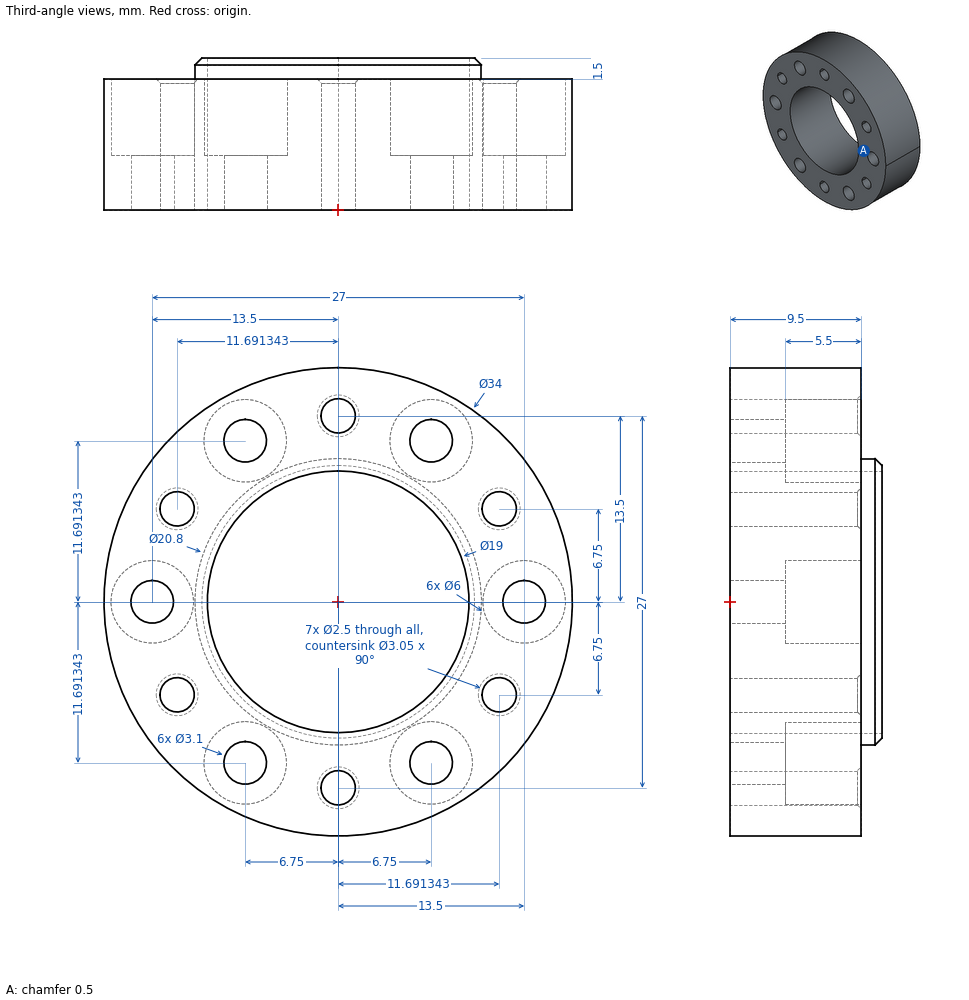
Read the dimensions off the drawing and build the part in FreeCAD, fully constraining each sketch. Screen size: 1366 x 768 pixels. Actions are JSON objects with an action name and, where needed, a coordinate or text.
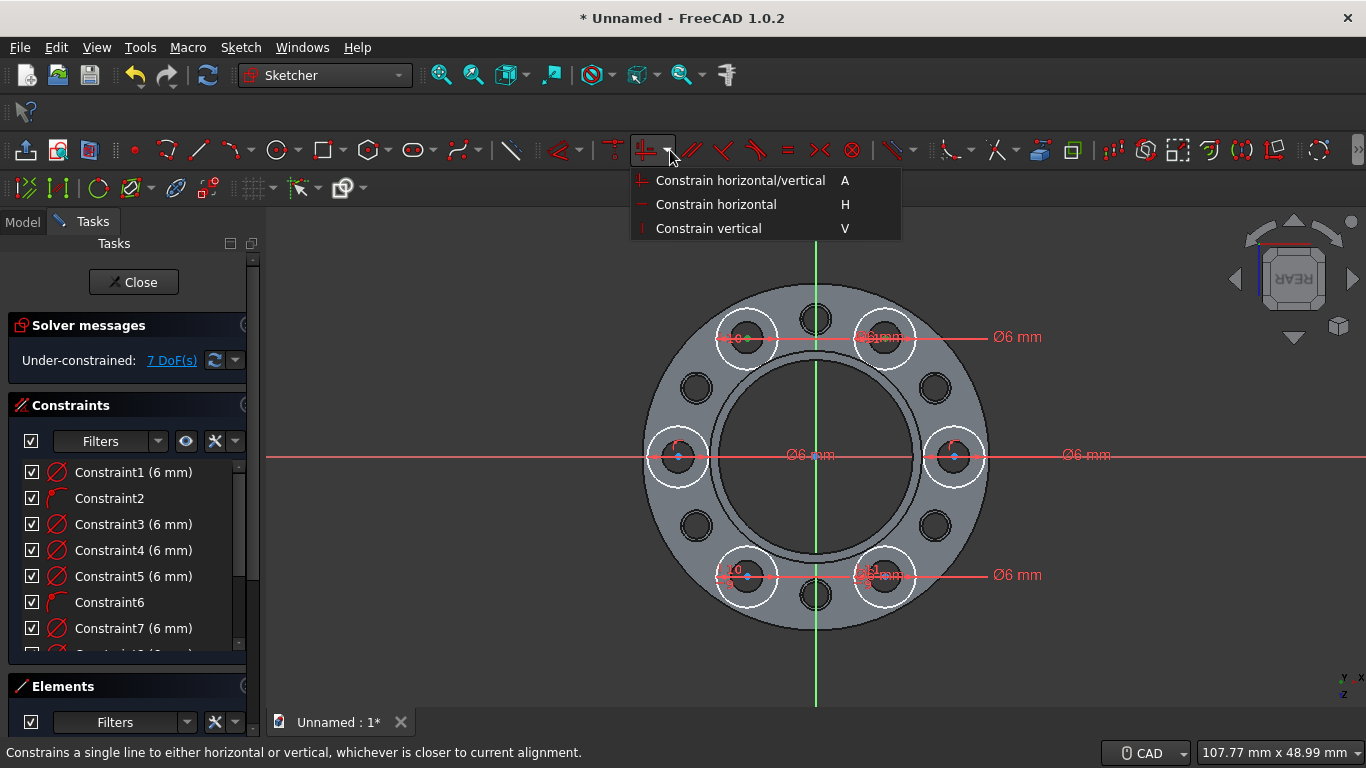
{"action": "left_click", "coordinate": [766, 204]}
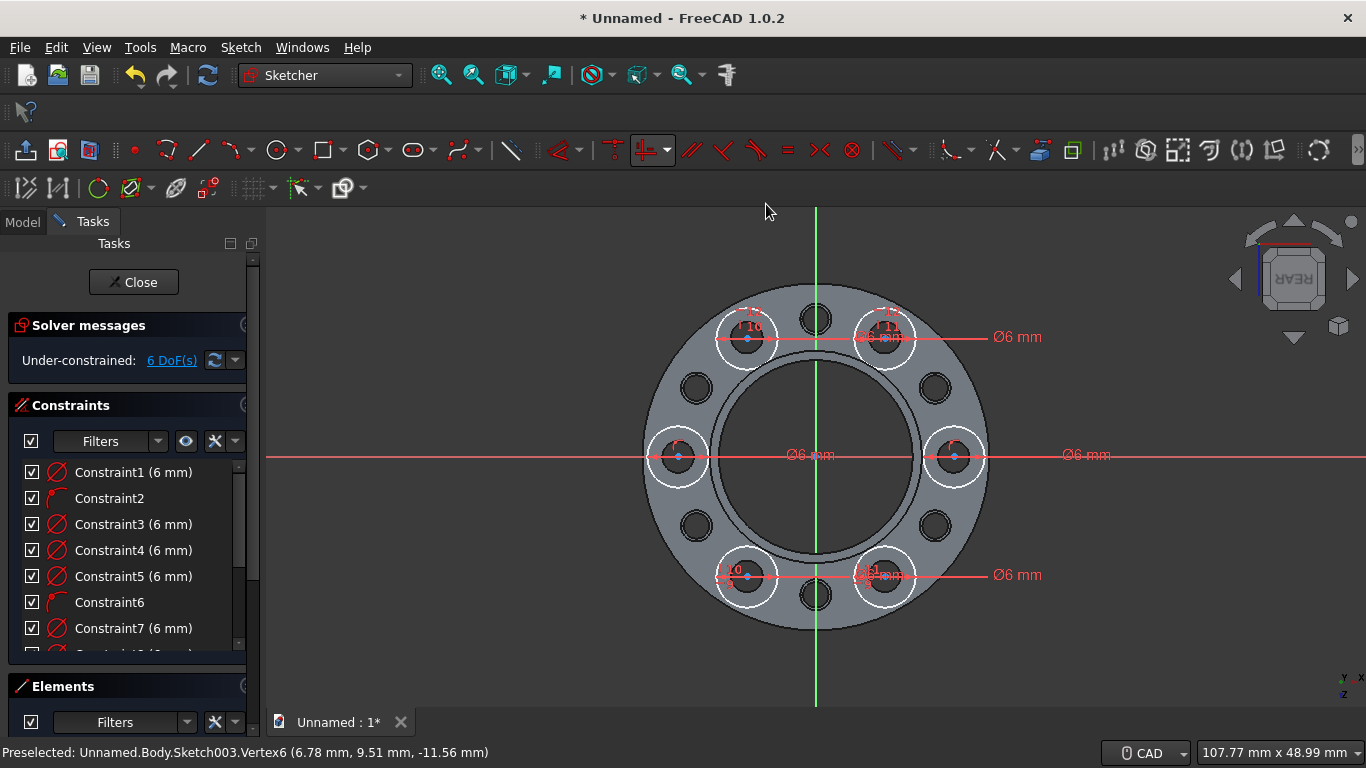
{"action": "left_click", "coordinate": [558, 150]}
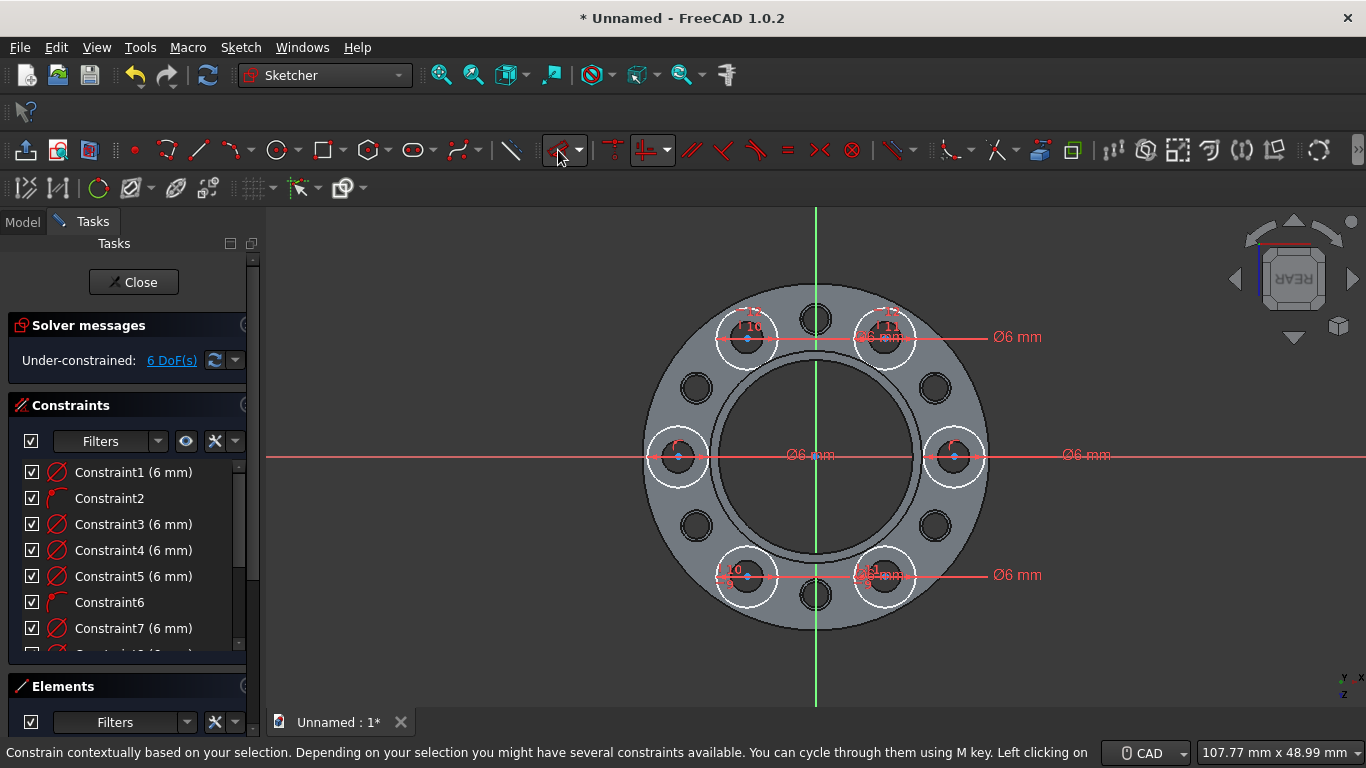
{"action": "left_click", "coordinate": [954, 457]}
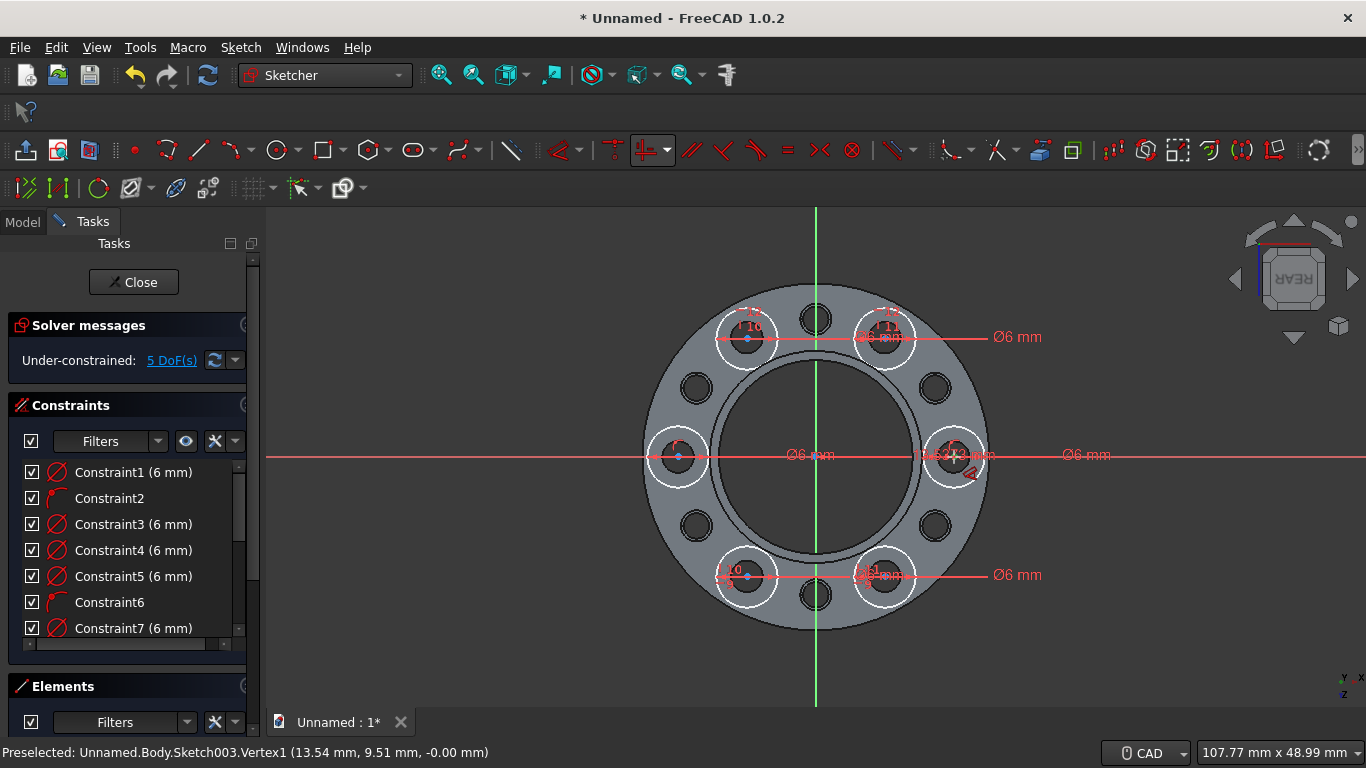
{"action": "left_click", "coordinate": [678, 457]}
{"action": "left_click", "coordinate": [753, 491]}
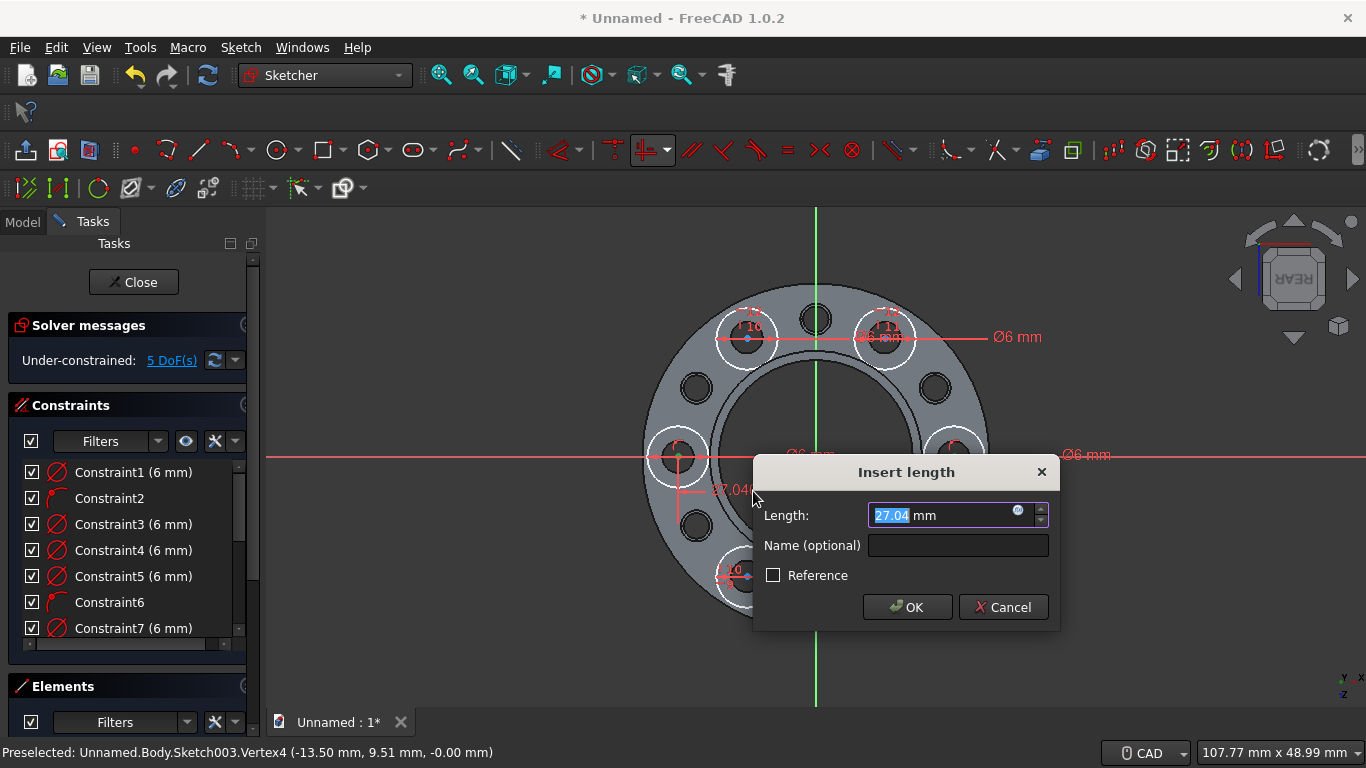
{"action": "type", "text": "27"}
{"action": "key", "text": "Return"}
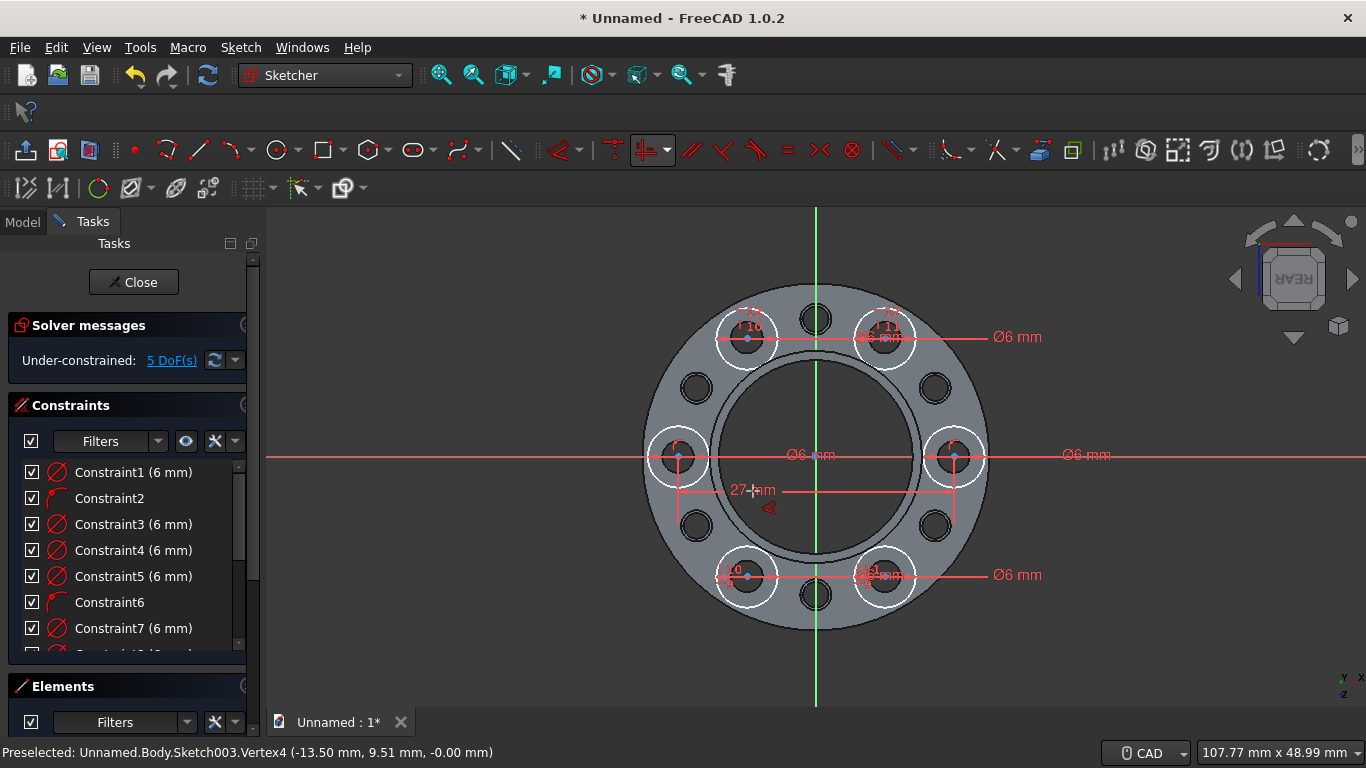
{"action": "left_click", "coordinate": [954, 457]}
{"action": "left_click", "coordinate": [885, 491]}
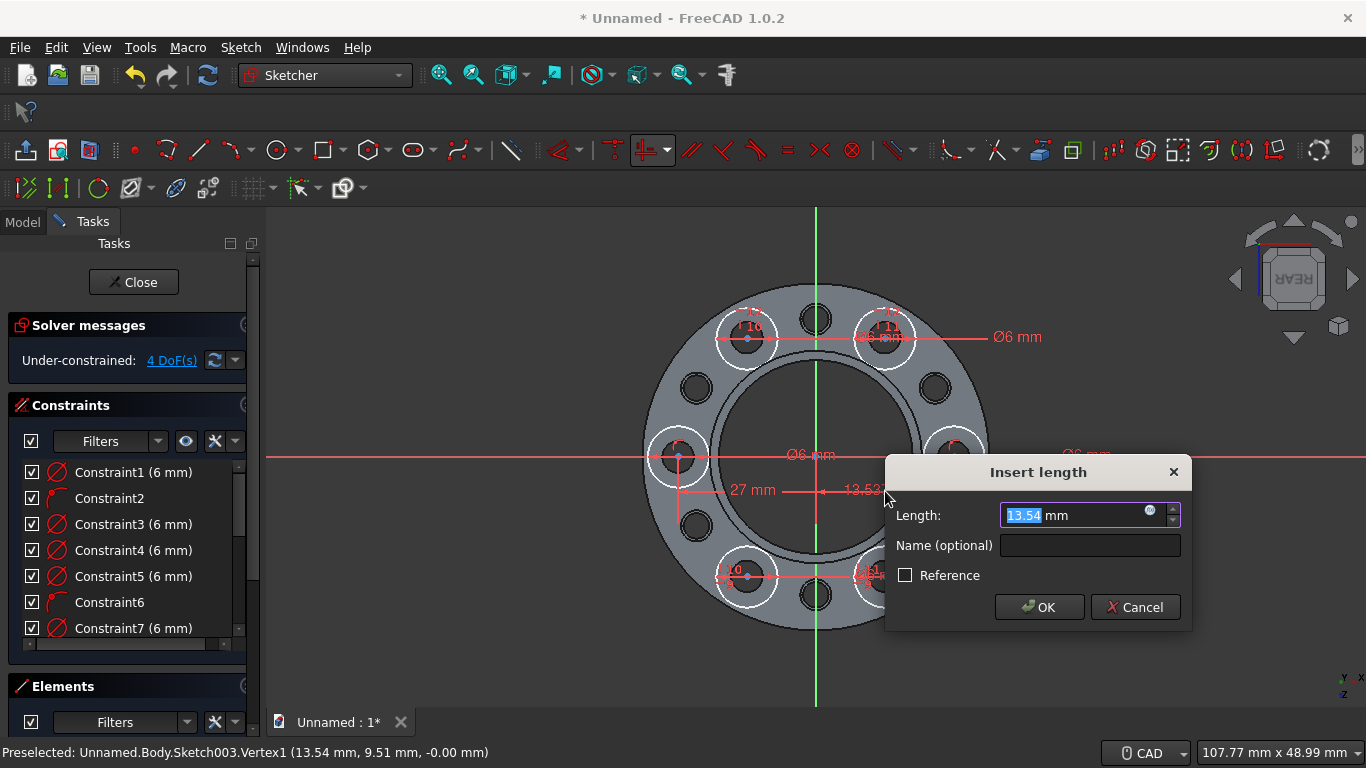
{"action": "type", "text": "13.5"}
{"action": "key", "text": "Return"}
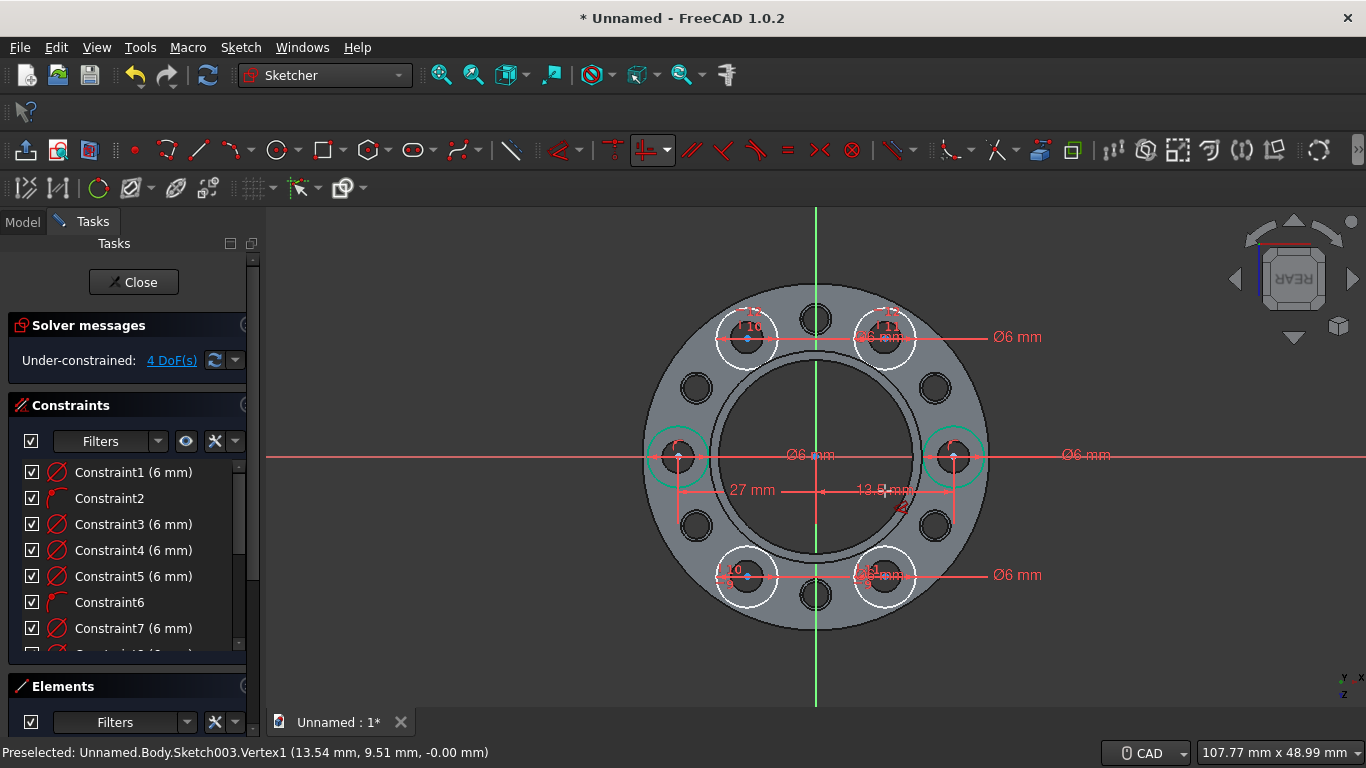
{"action": "left_click", "coordinate": [885, 577]}
{"action": "left_click", "coordinate": [850, 611]}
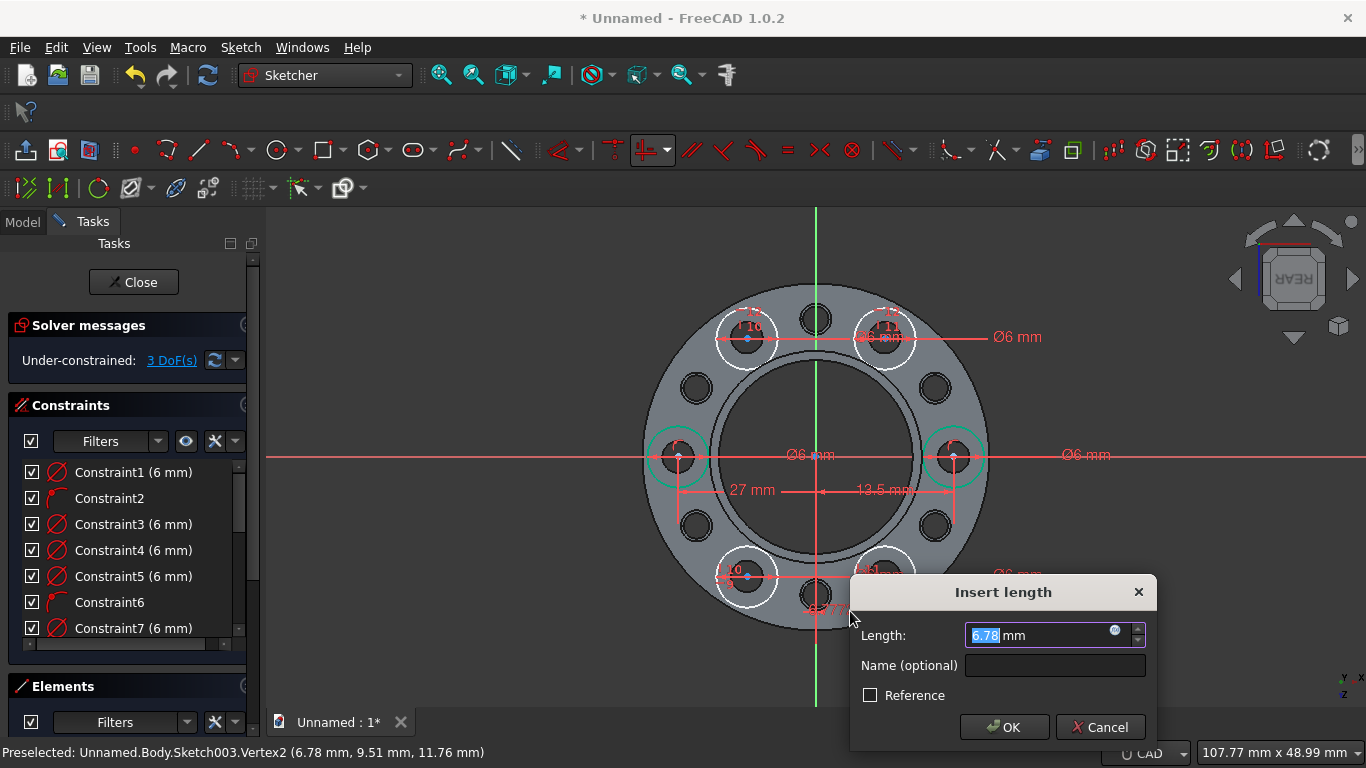
{"action": "type", "text": "6.75"}
{"action": "key", "text": "Return"}